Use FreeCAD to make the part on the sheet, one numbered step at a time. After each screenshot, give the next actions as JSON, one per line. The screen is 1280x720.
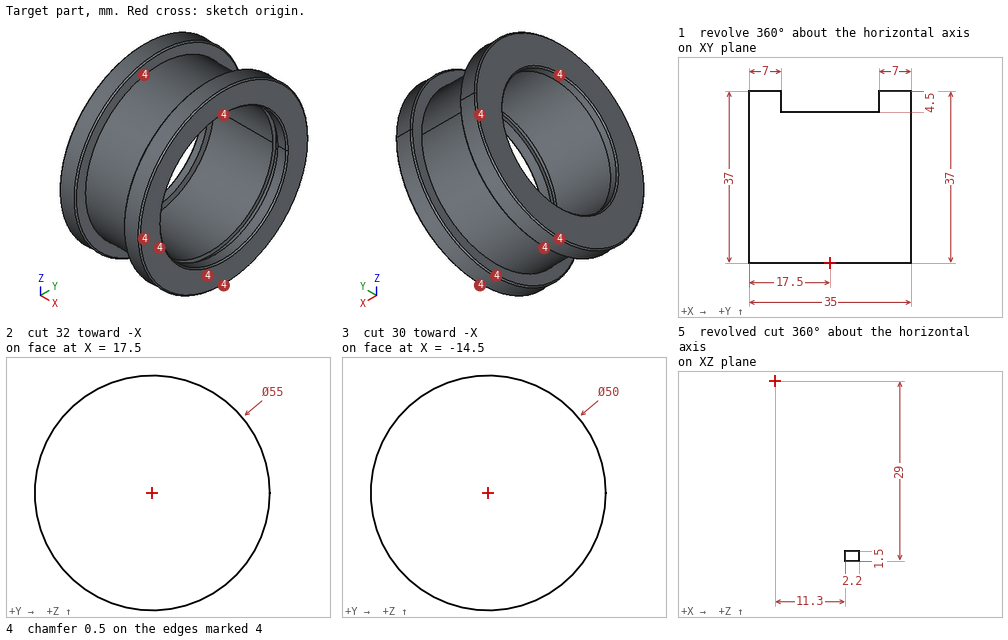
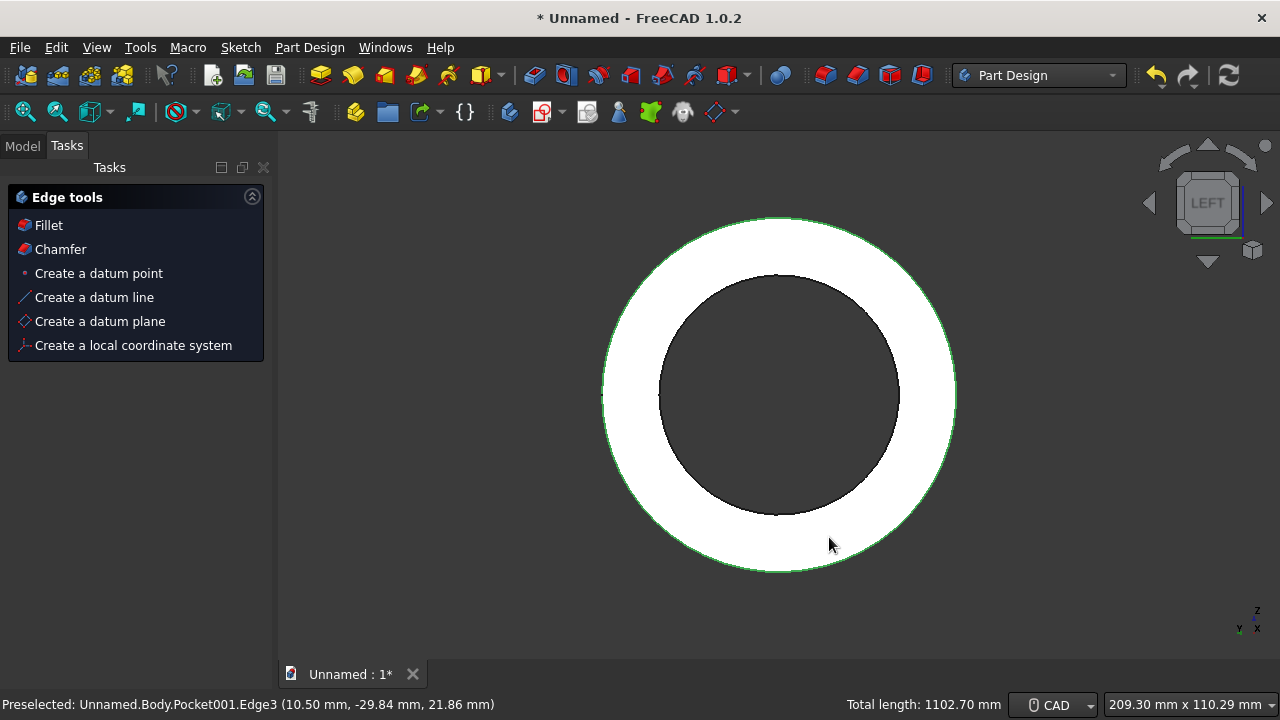
{"action": "left_click", "coordinate": [899, 394], "text": "ctrl"}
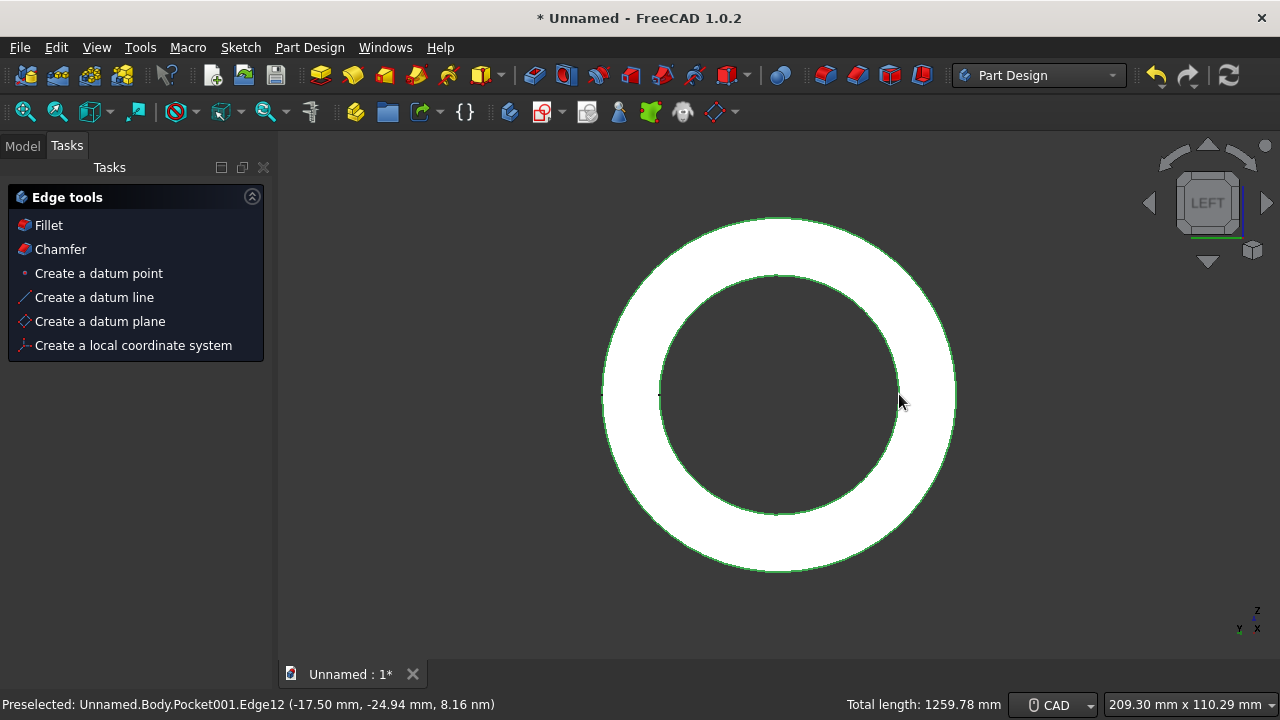
{"action": "left_click", "coordinate": [858, 76]}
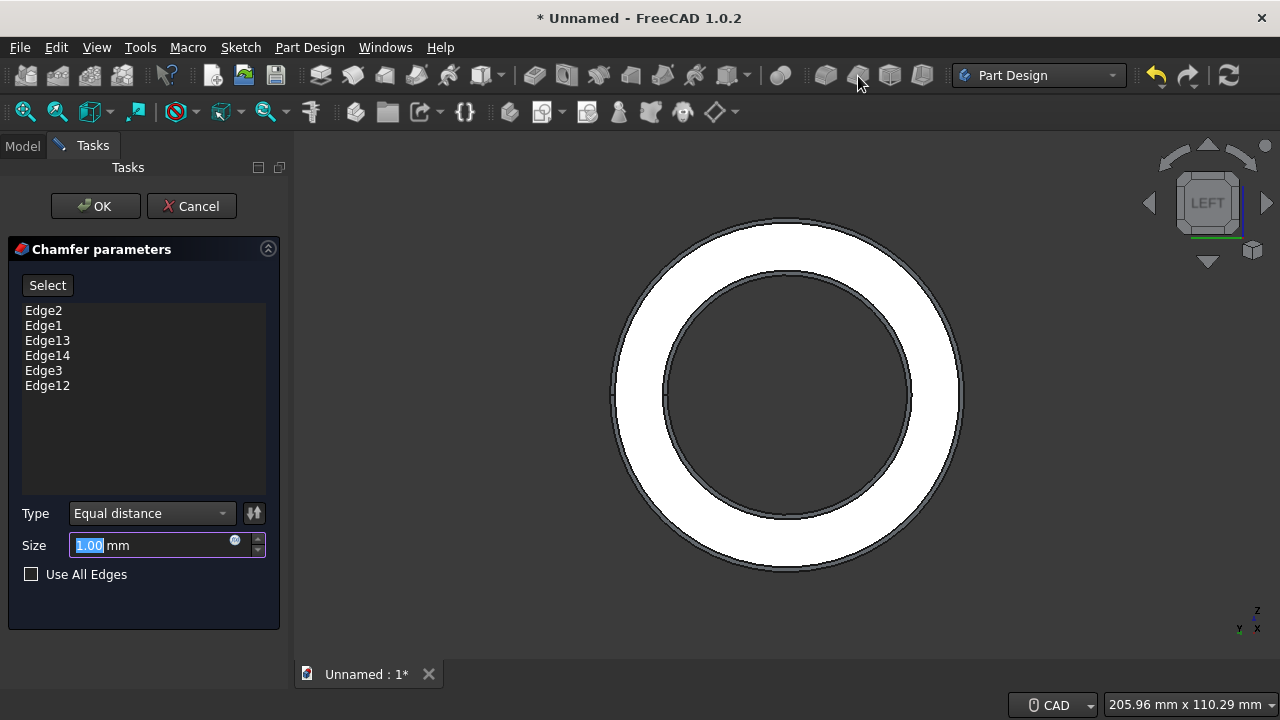
{"action": "type", "text": "0.5"}
{"action": "key", "text": "Tab"}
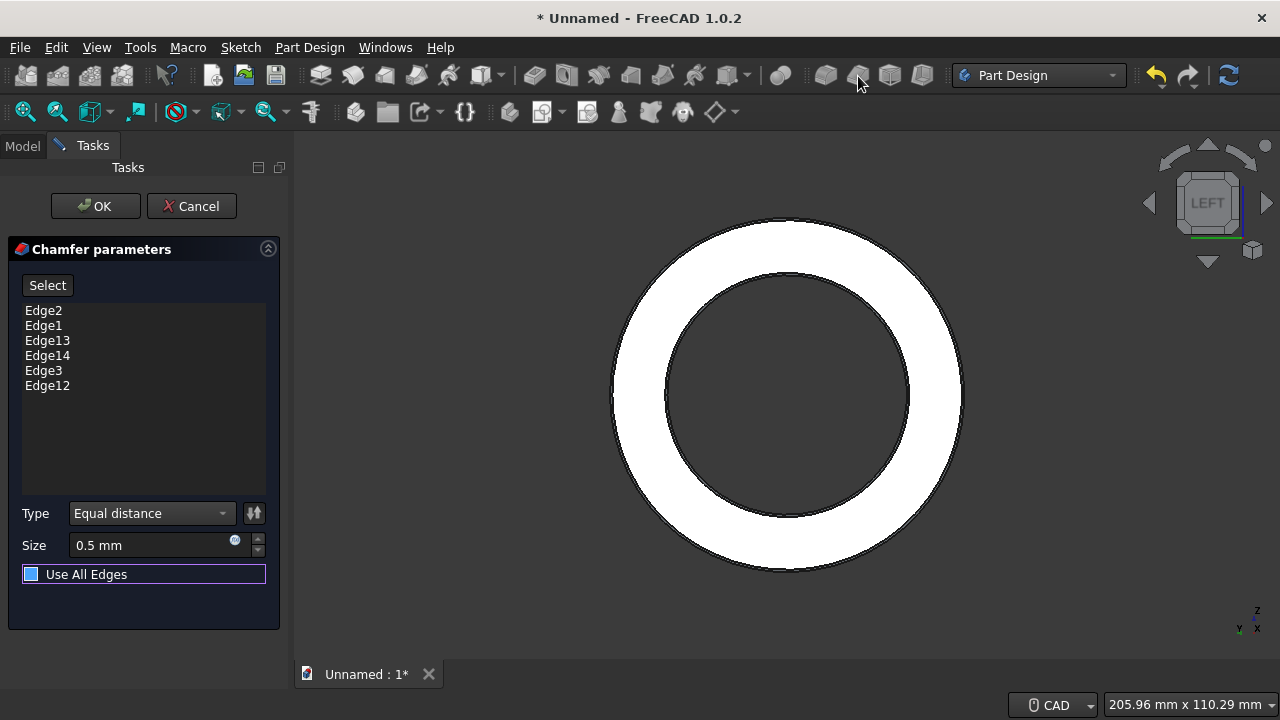
{"action": "left_click", "coordinate": [96, 206]}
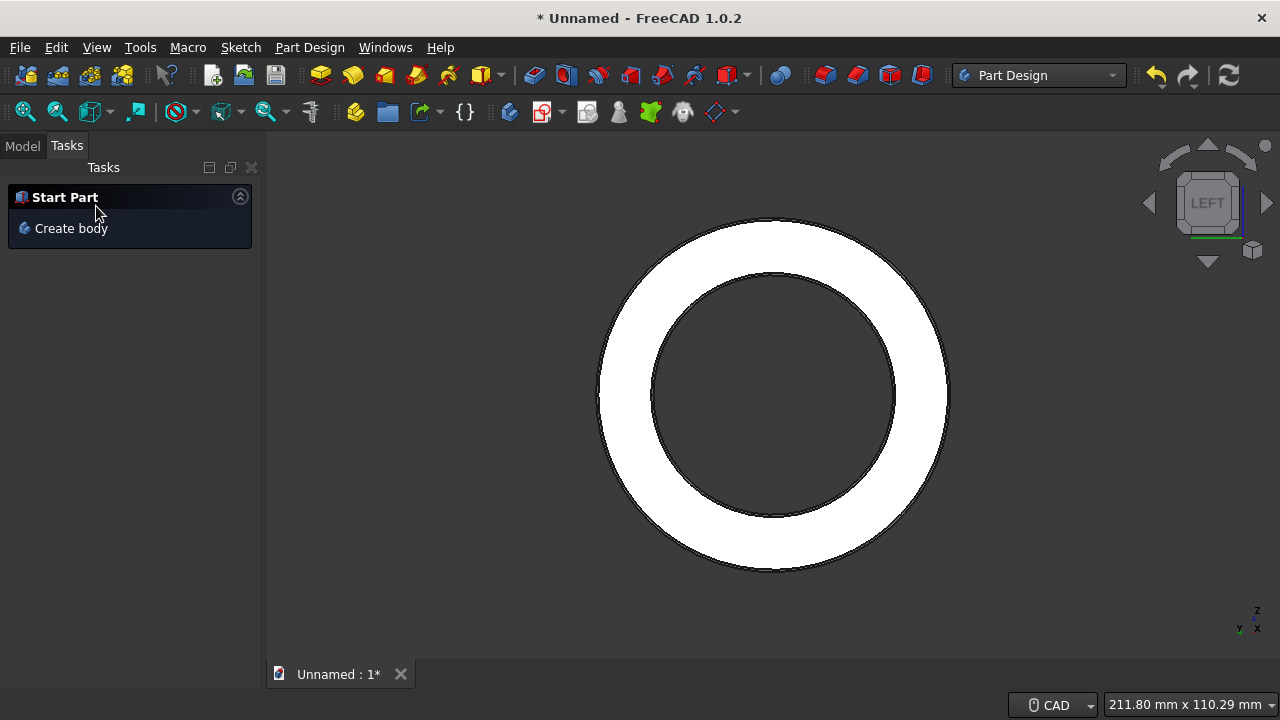
{"action": "left_click", "coordinate": [542, 112]}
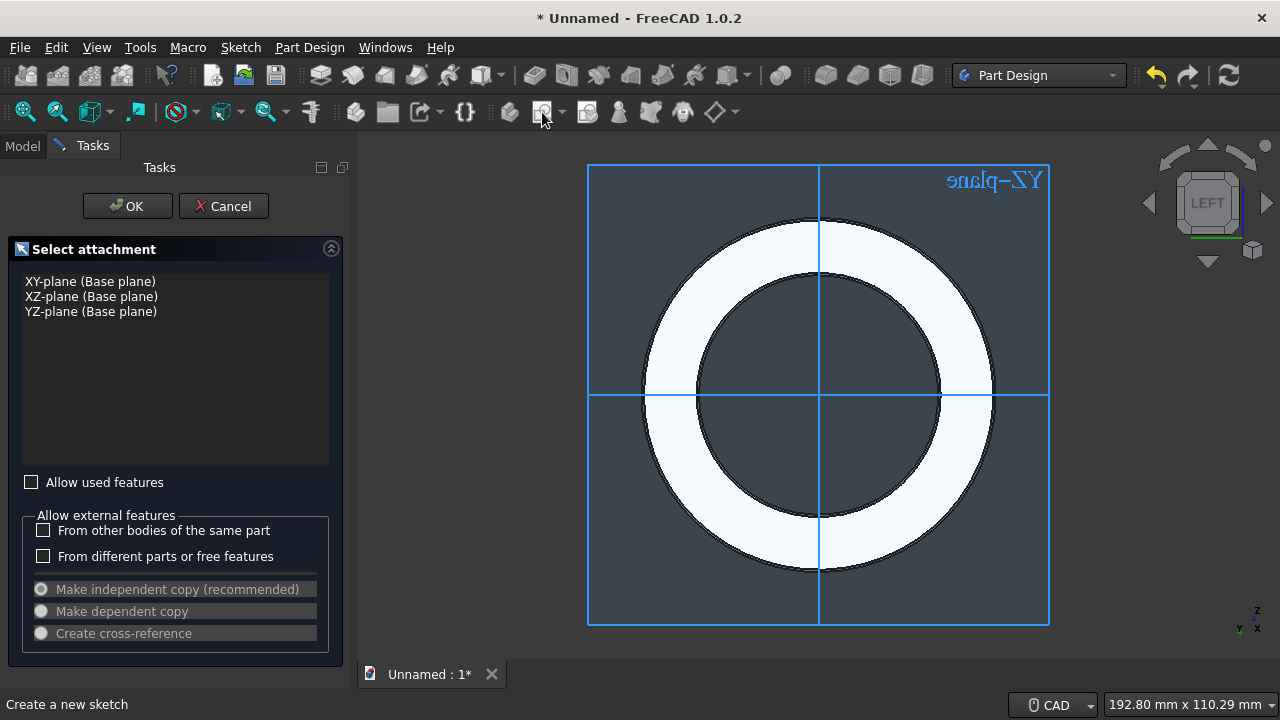
{"action": "left_click", "coordinate": [82, 296]}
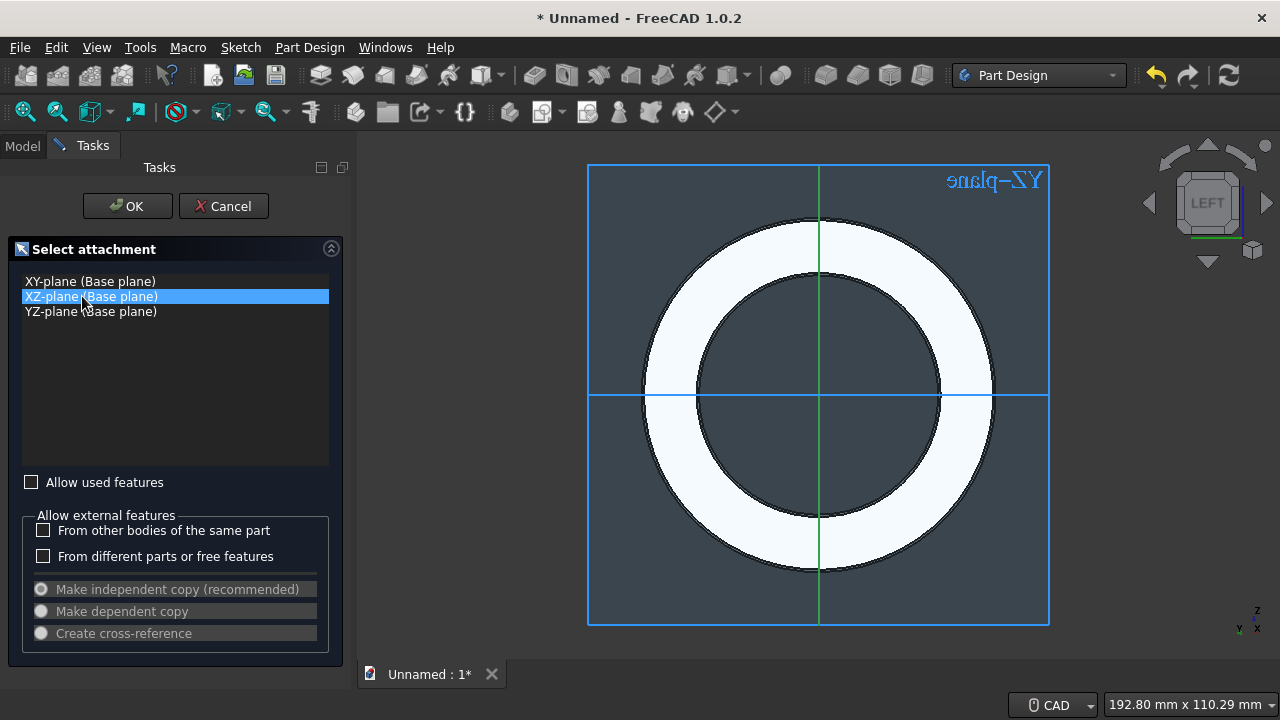
{"action": "left_click", "coordinate": [128, 206]}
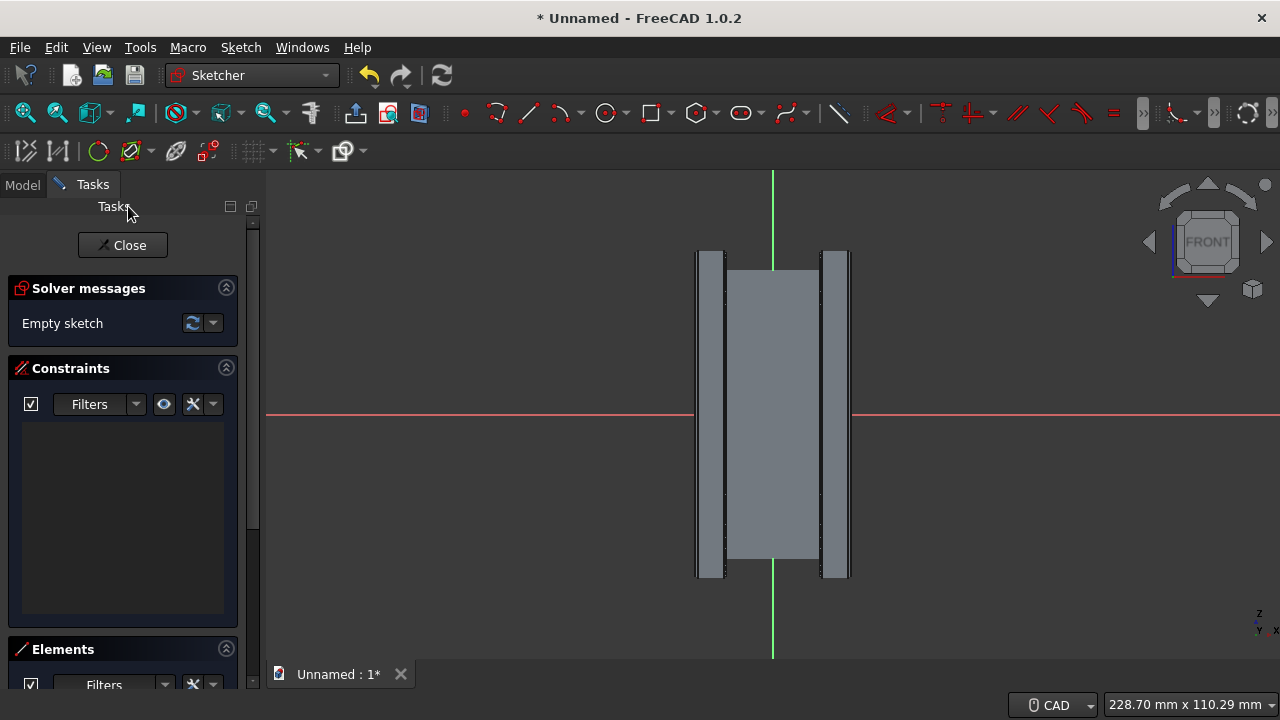
{"action": "left_click", "coordinate": [420, 114]}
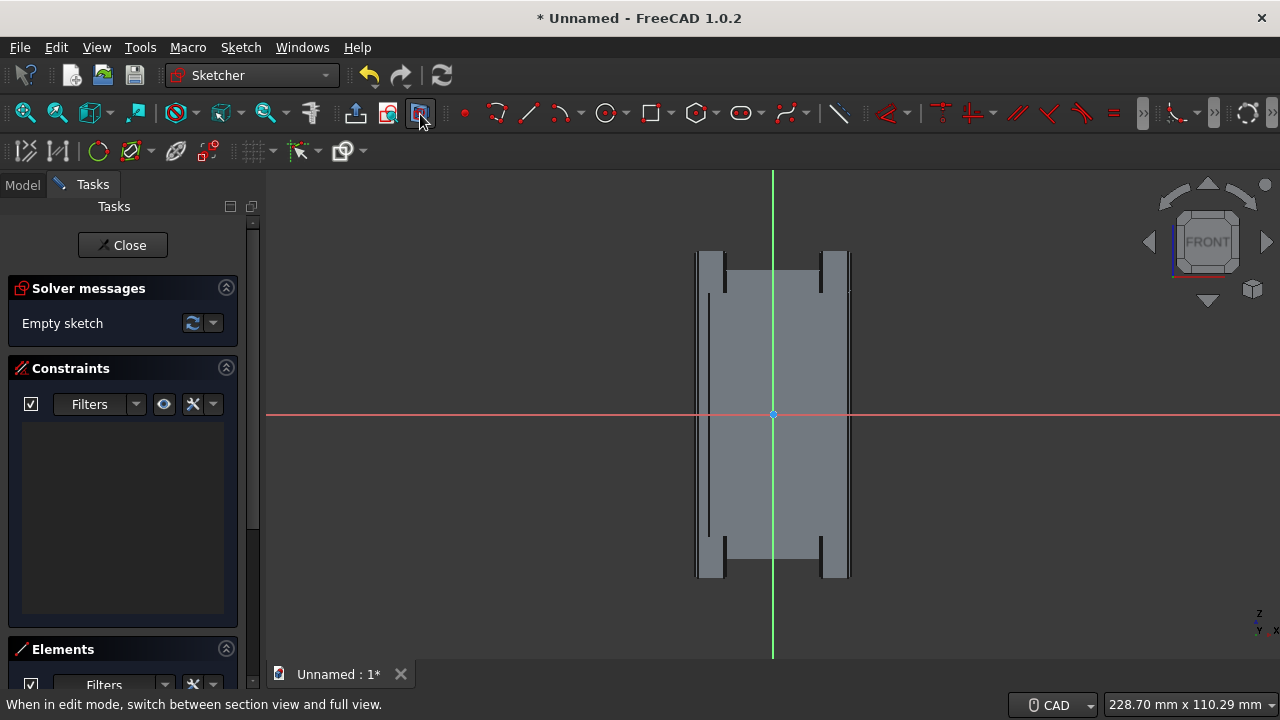
{"action": "scroll", "coordinate": [834, 546], "scroll_direction": "up", "scroll_amount": 15}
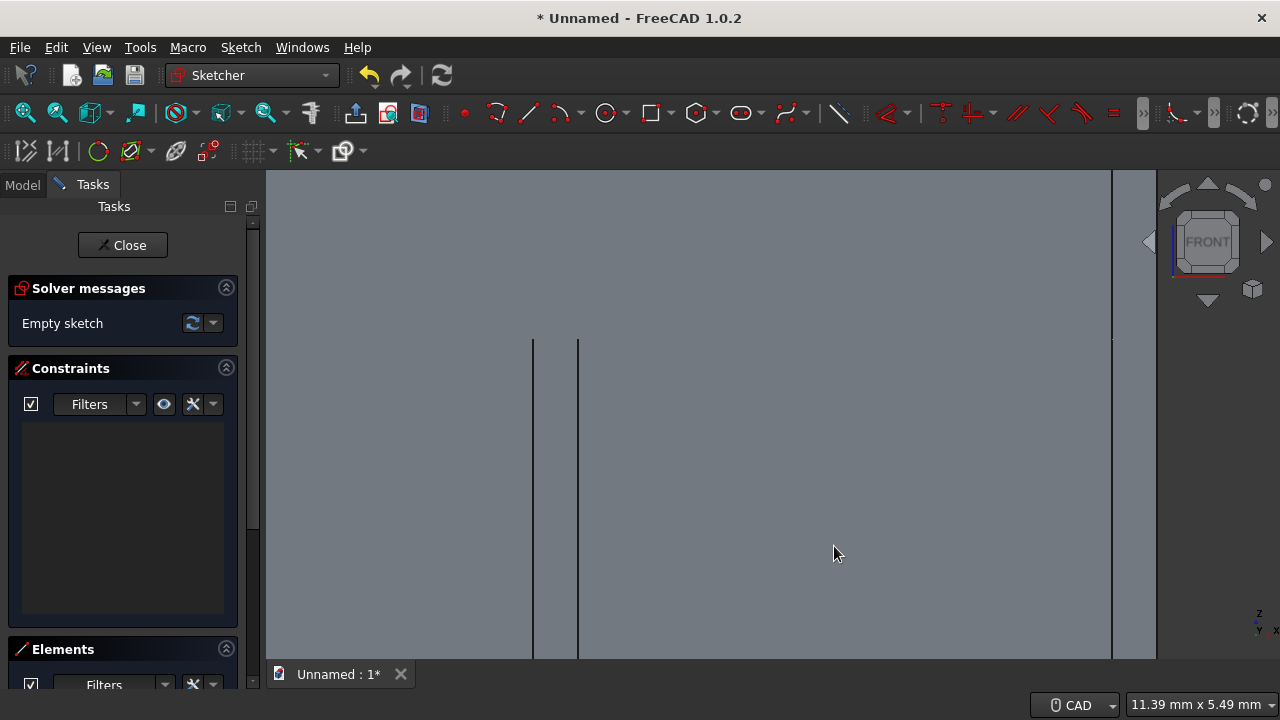
{"action": "scroll", "coordinate": [701, 399], "scroll_direction": "up", "scroll_amount": 4}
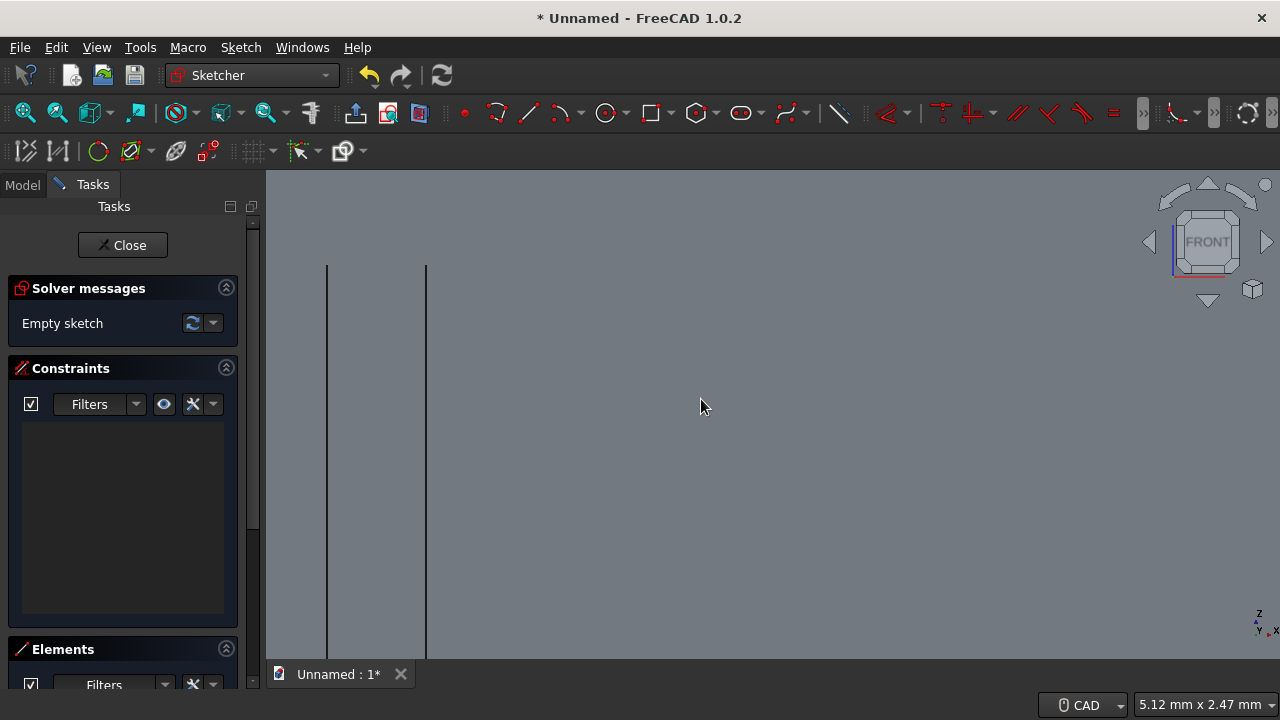
{"action": "left_click", "coordinate": [652, 114]}